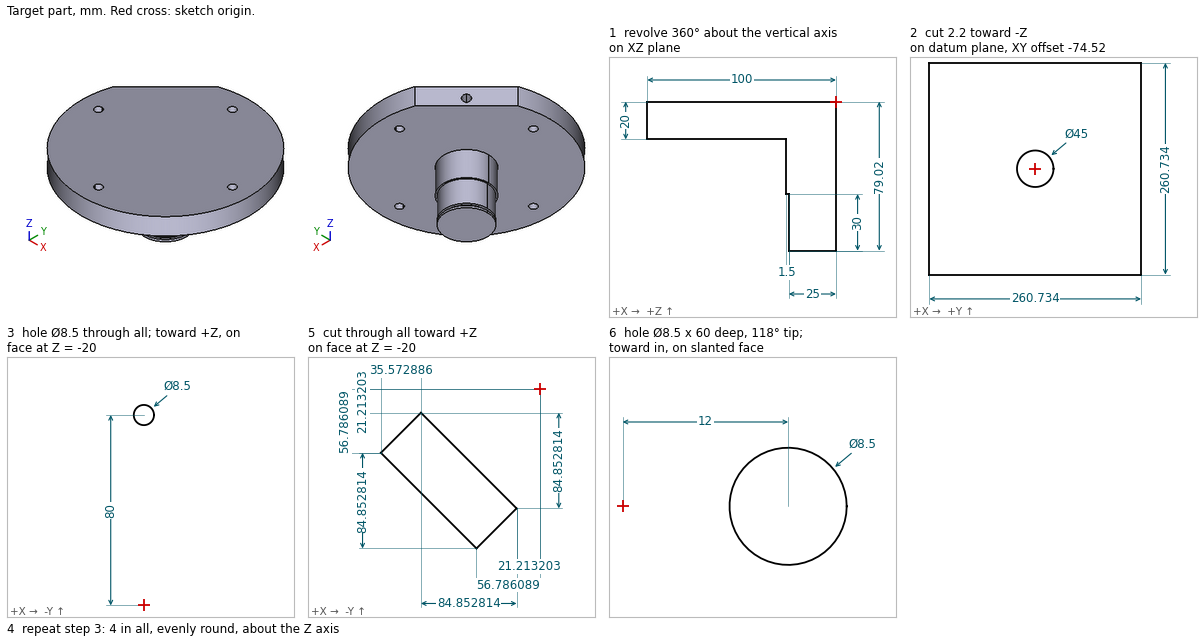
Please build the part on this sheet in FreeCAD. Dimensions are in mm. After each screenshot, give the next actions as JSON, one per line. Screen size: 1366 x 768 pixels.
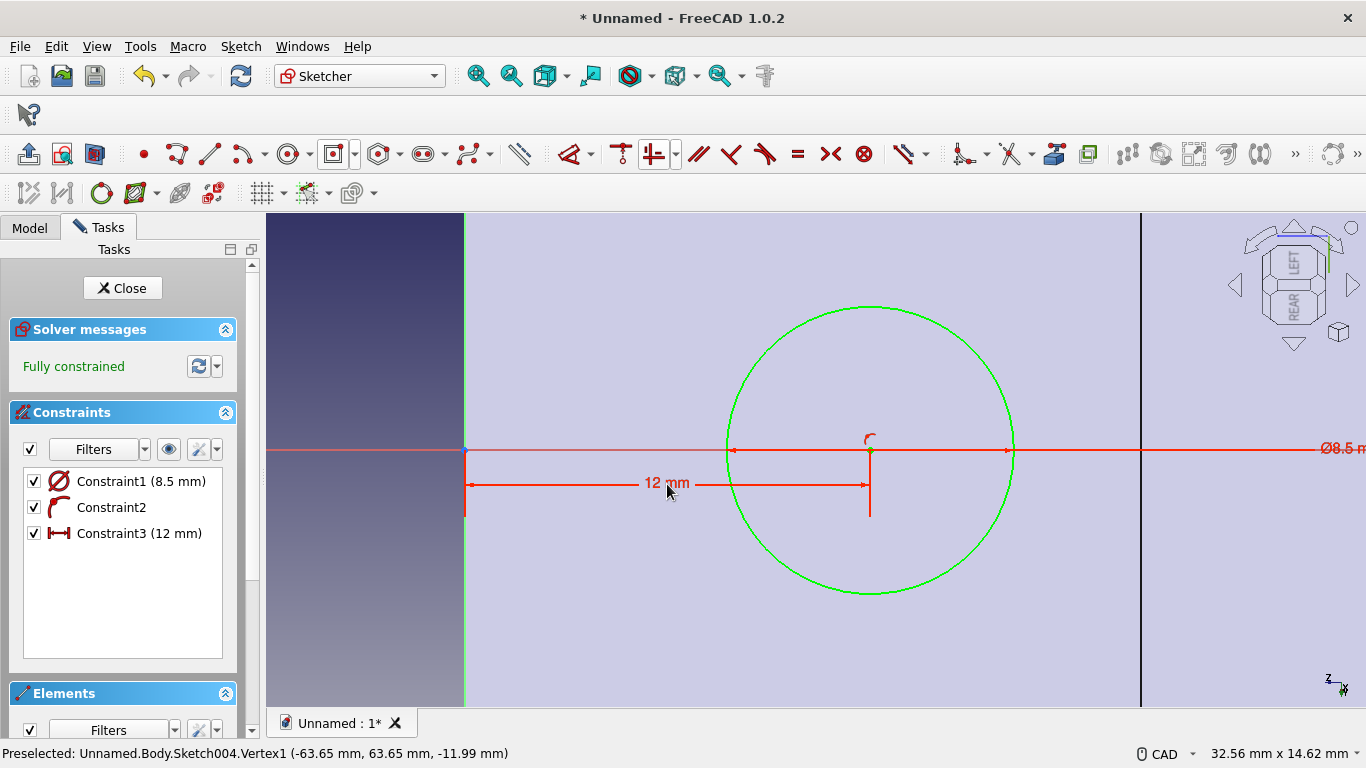
{"action": "left_click", "coordinate": [123, 288]}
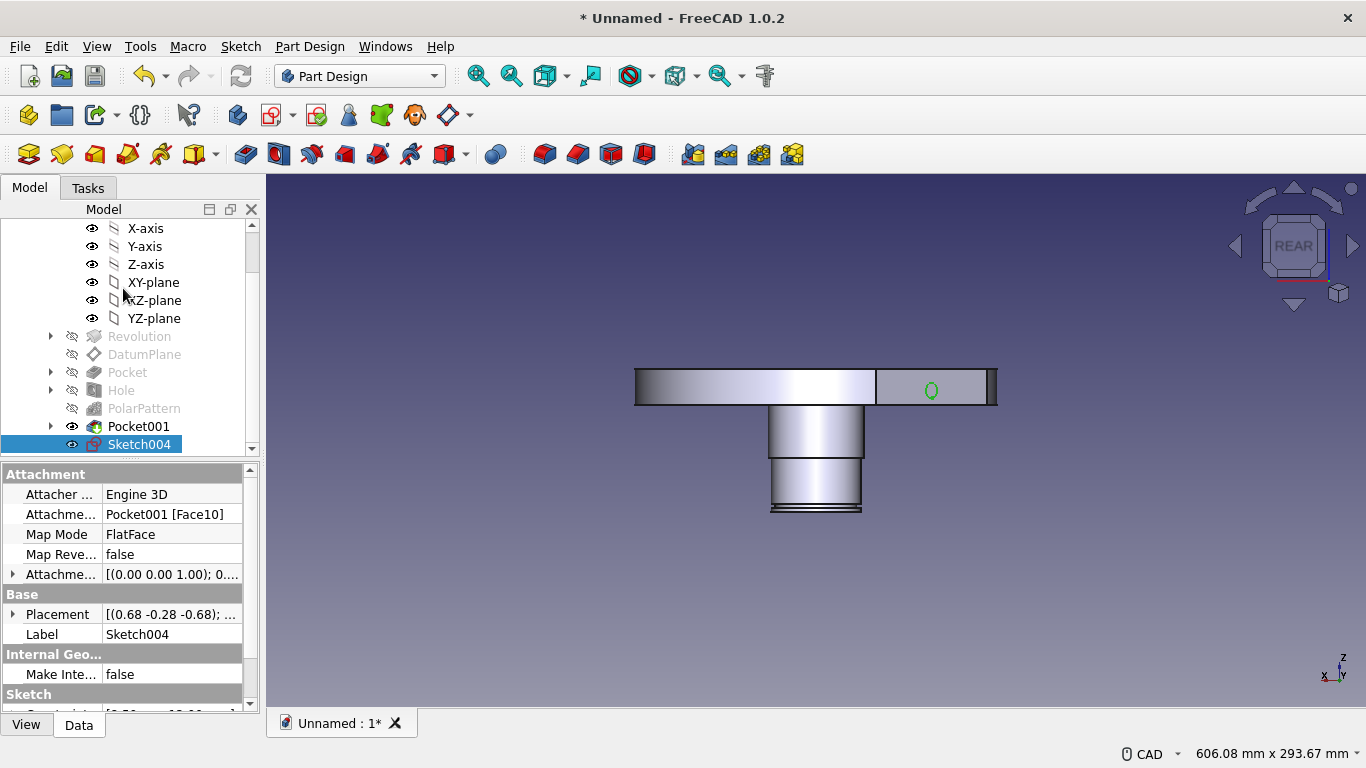
{"action": "left_click", "coordinate": [279, 154]}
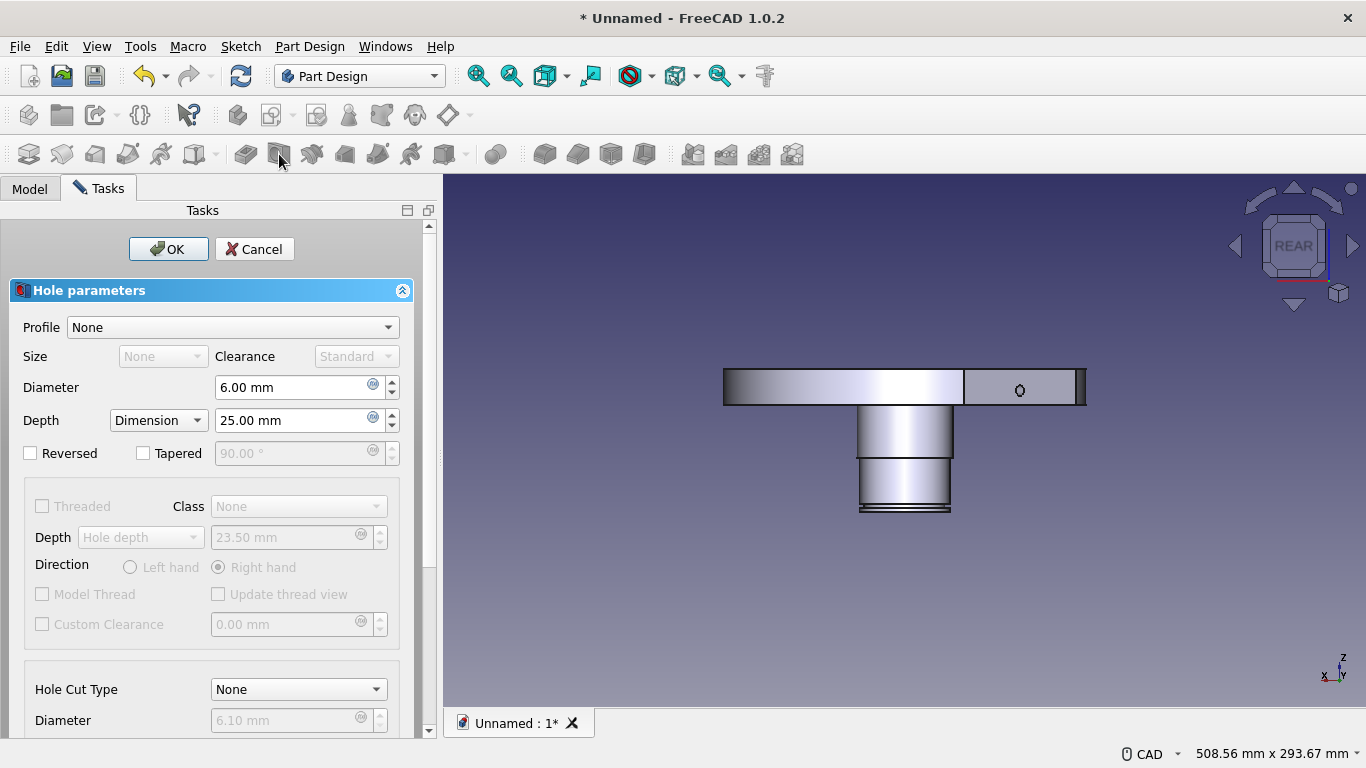
{"action": "triple_click", "coordinate": [300, 388]}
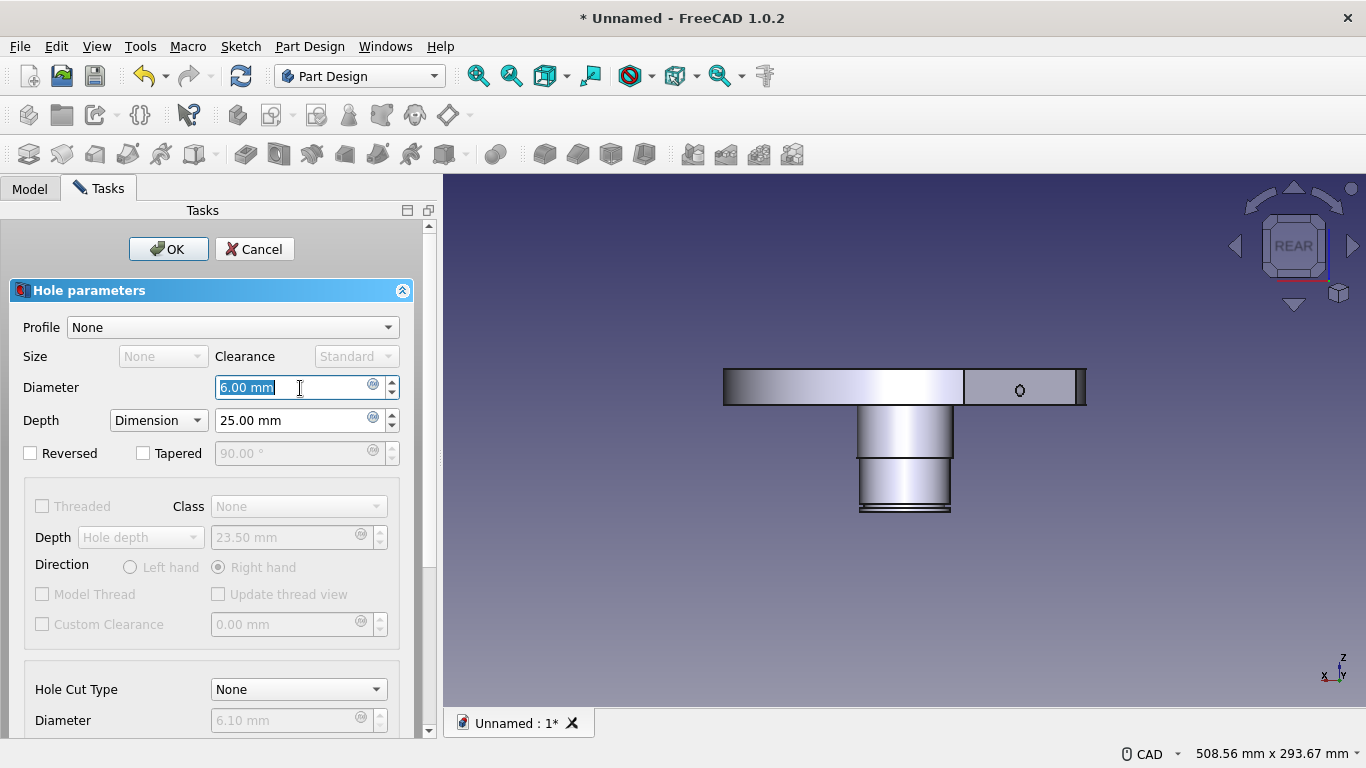
{"action": "type", "text": "8.5"}
{"action": "key", "text": "Tab"}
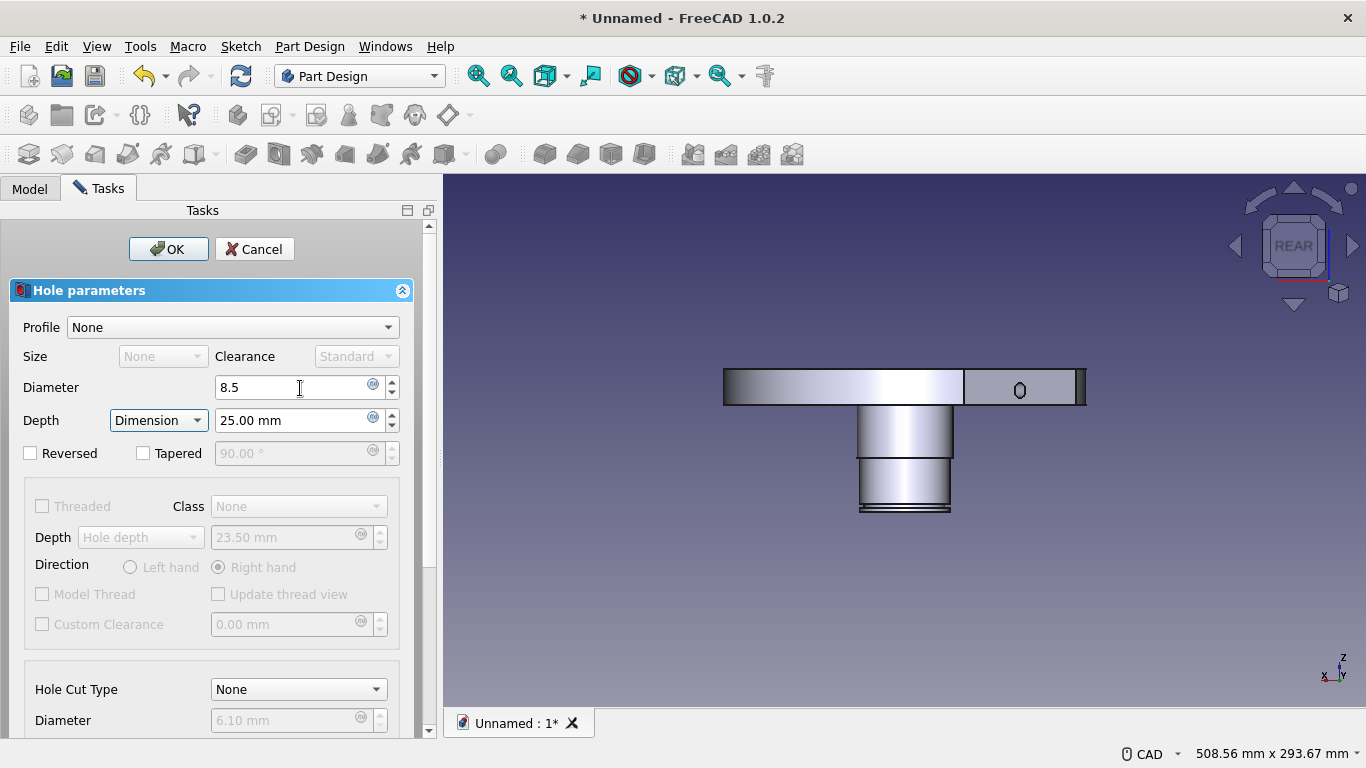
{"action": "triple_click", "coordinate": [300, 420]}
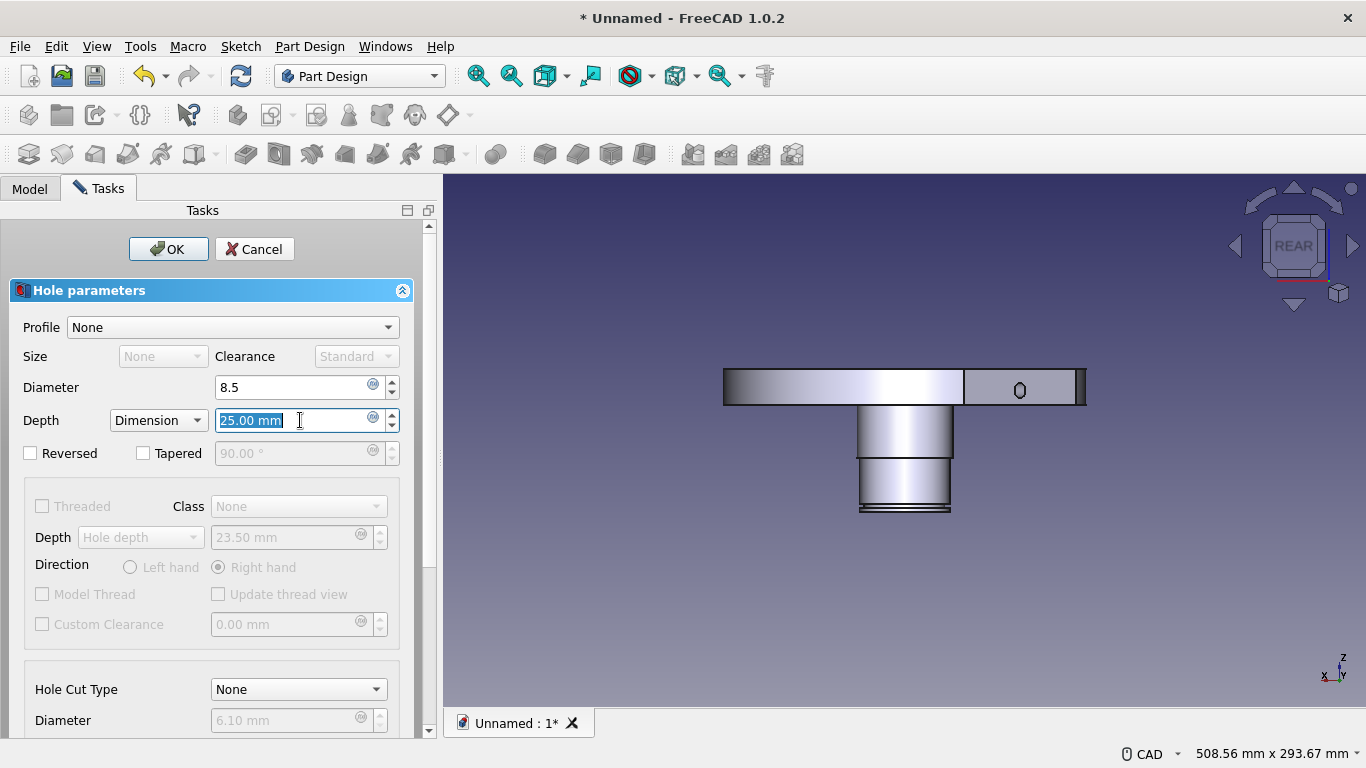
{"action": "type", "text": "60"}
{"action": "key", "text": "Tab"}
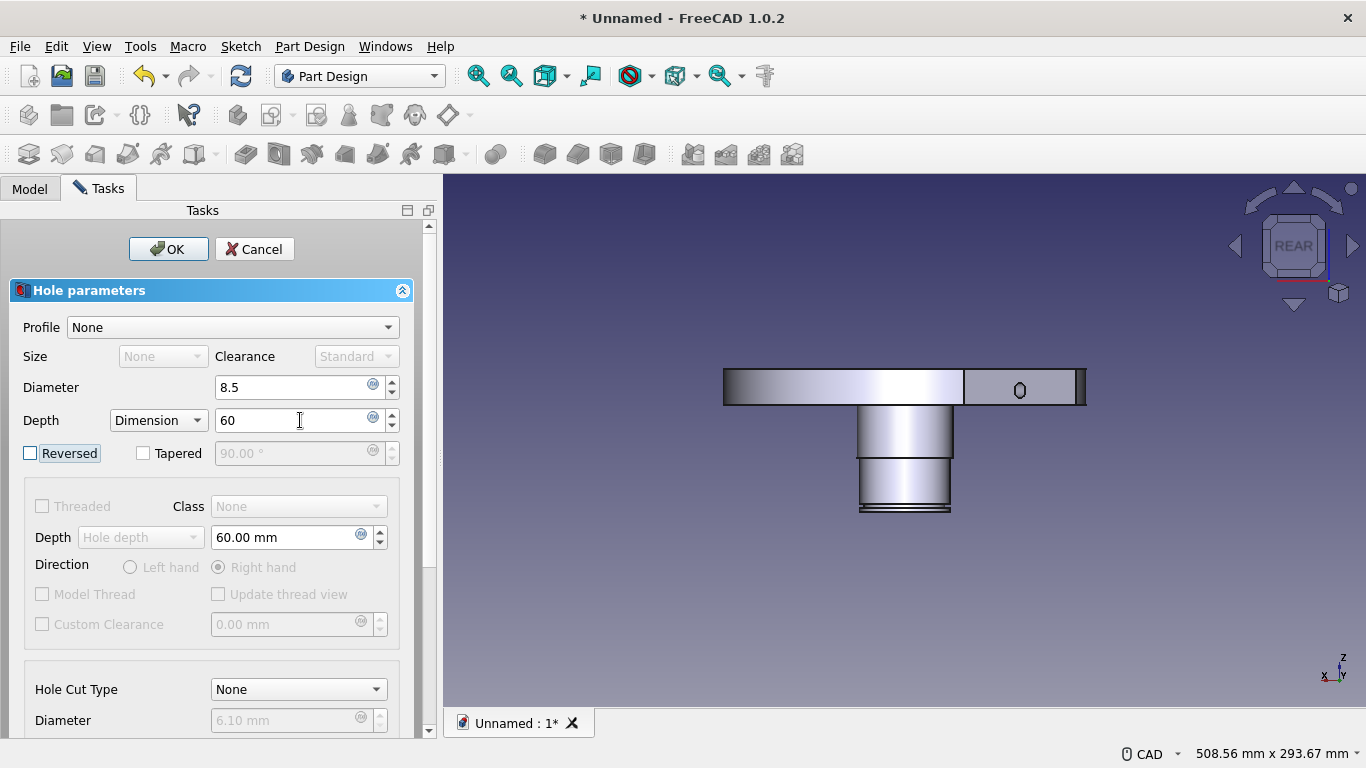
{"action": "left_click", "coordinate": [169, 249]}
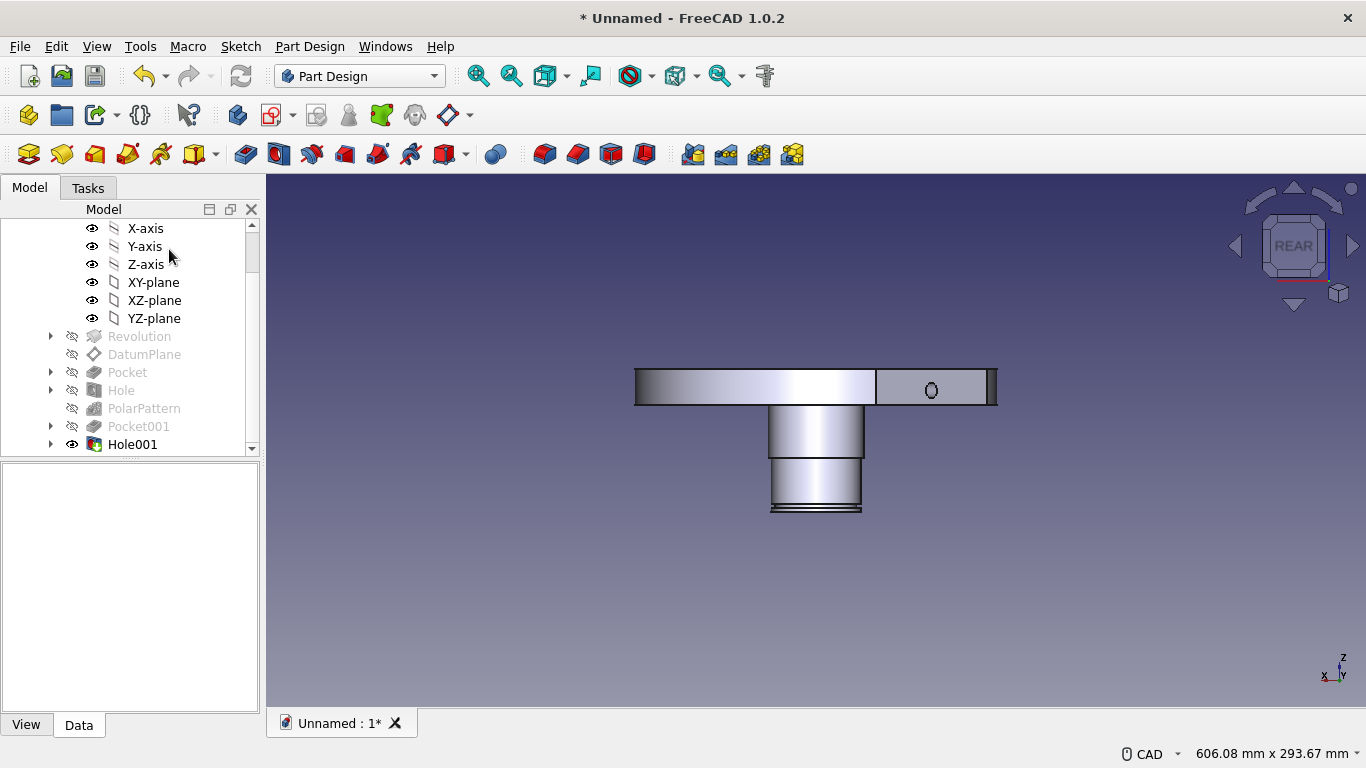
{"action": "key", "text": "0"}